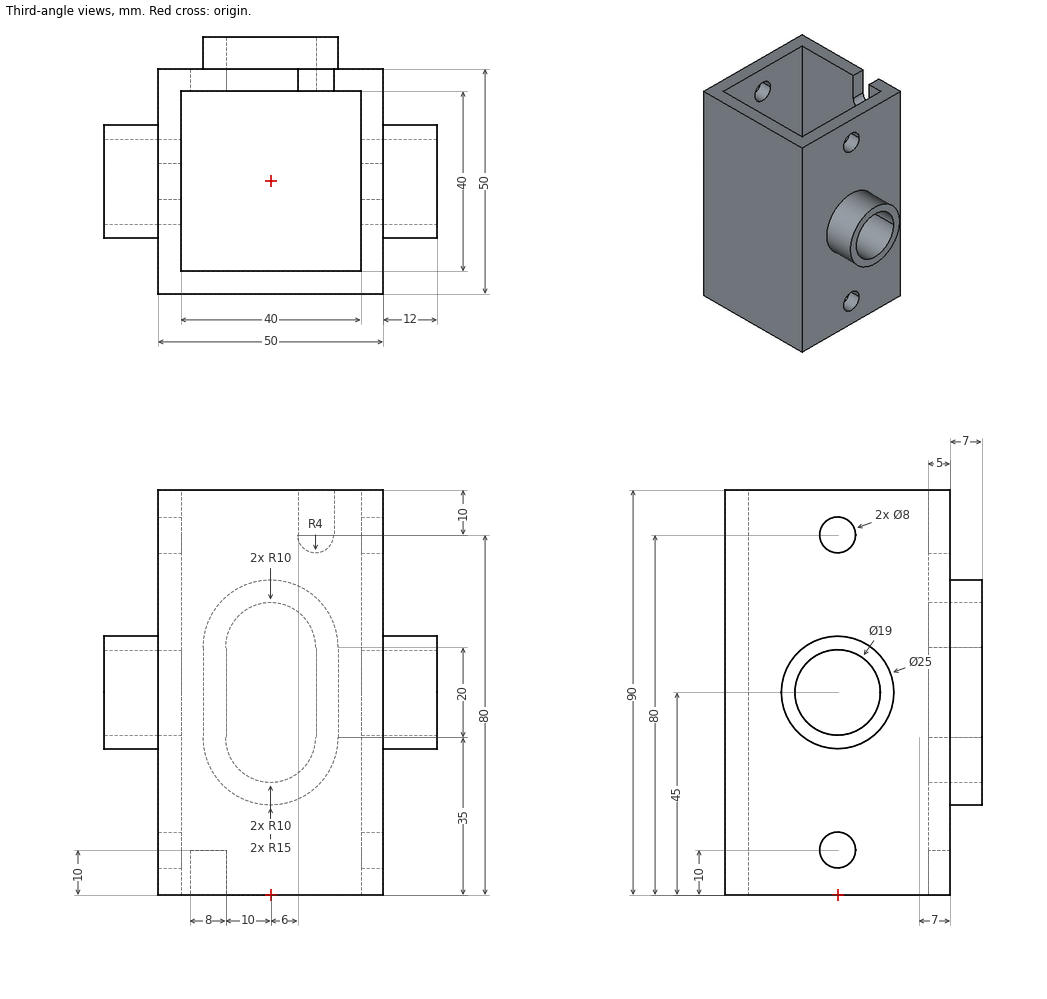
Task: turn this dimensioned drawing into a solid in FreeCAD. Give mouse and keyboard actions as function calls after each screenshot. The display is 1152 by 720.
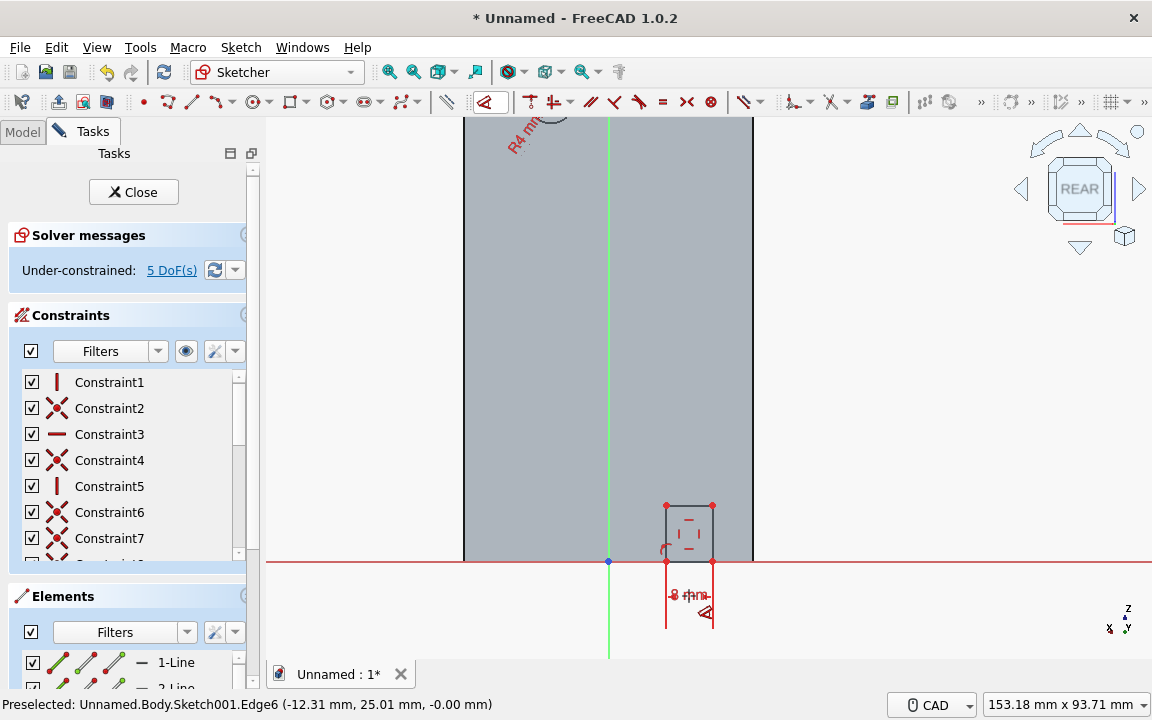
scroll(681, 564, down, 2)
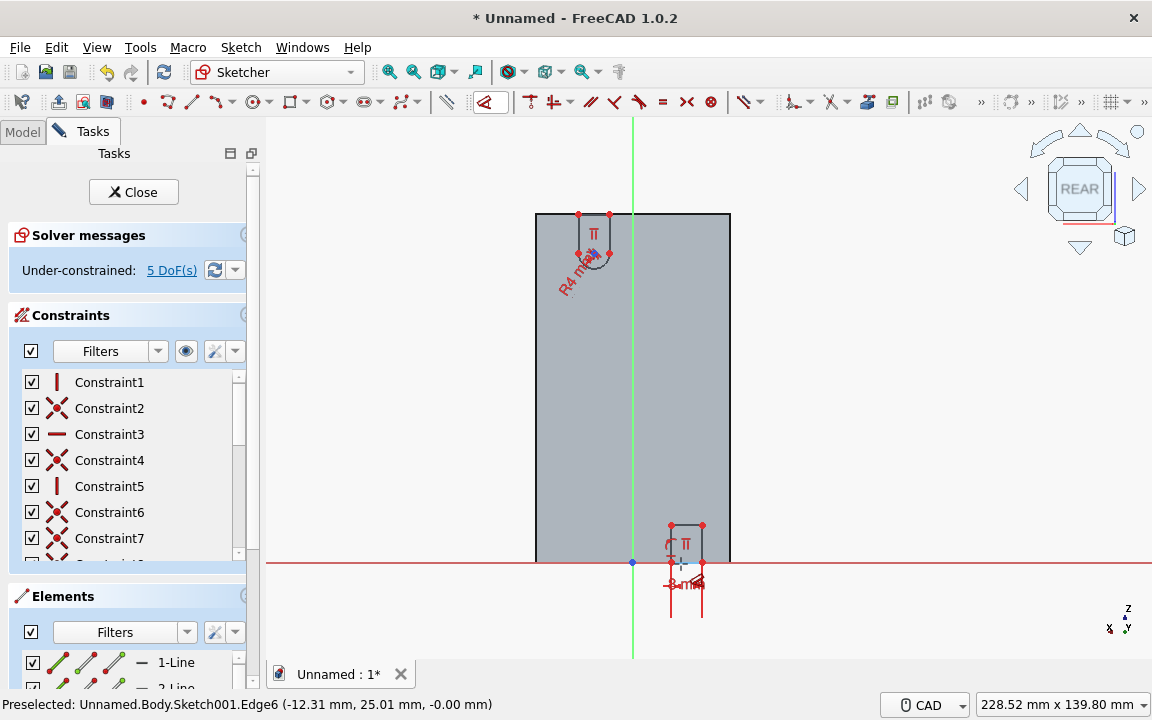
click(610, 242)
click(552, 234)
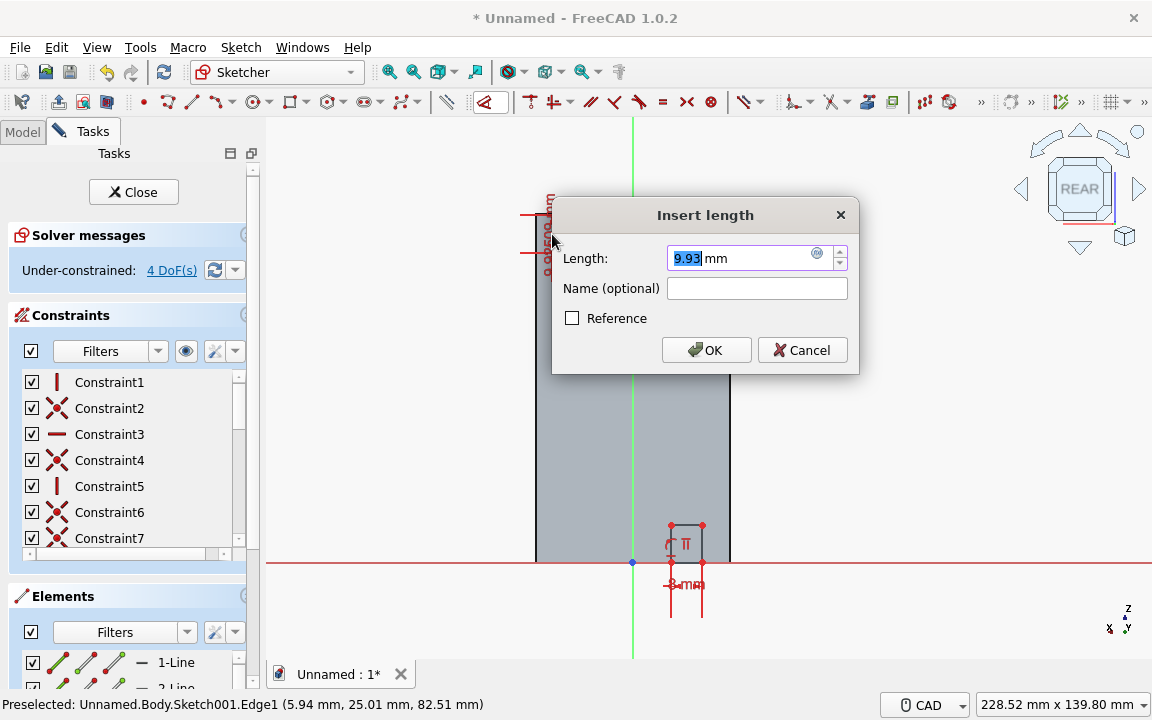
text(10)
key(Return)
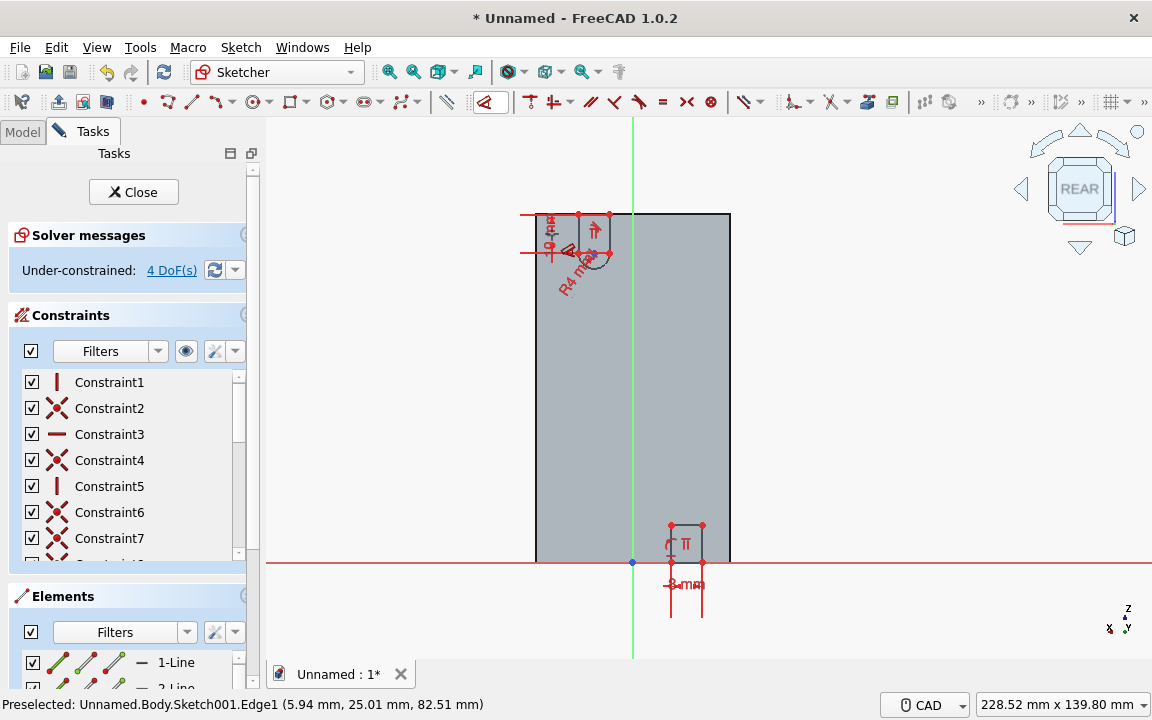
click(671, 536)
click(729, 544)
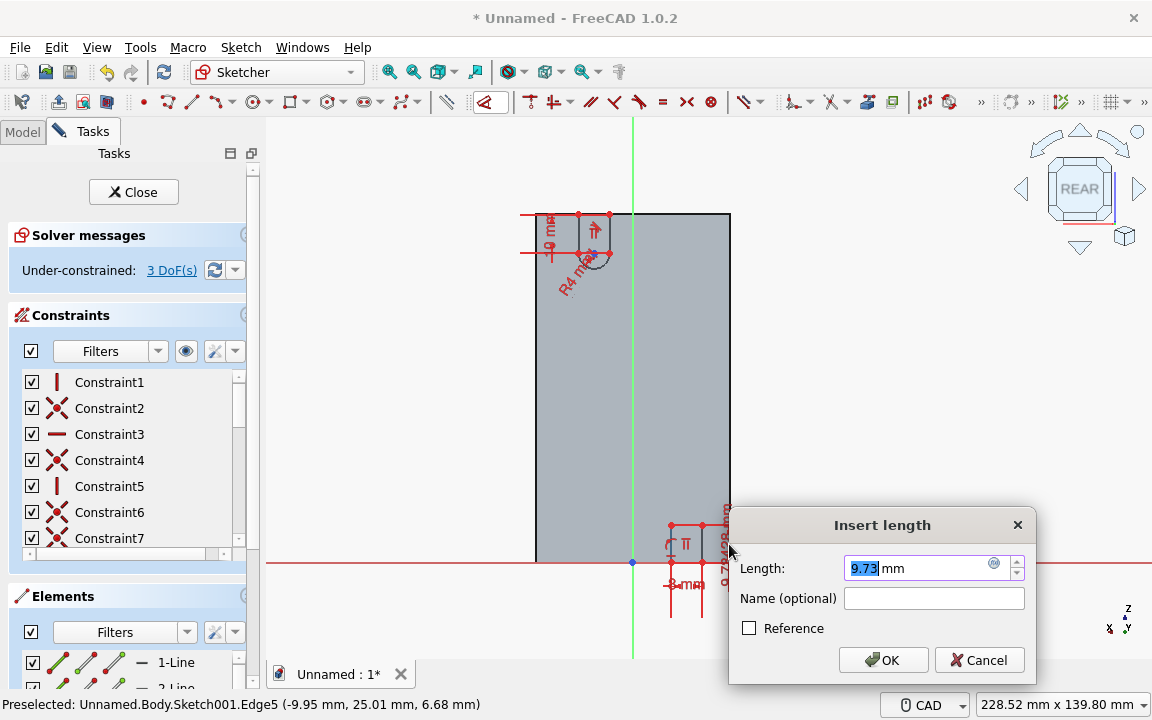
text(10)
key(Return)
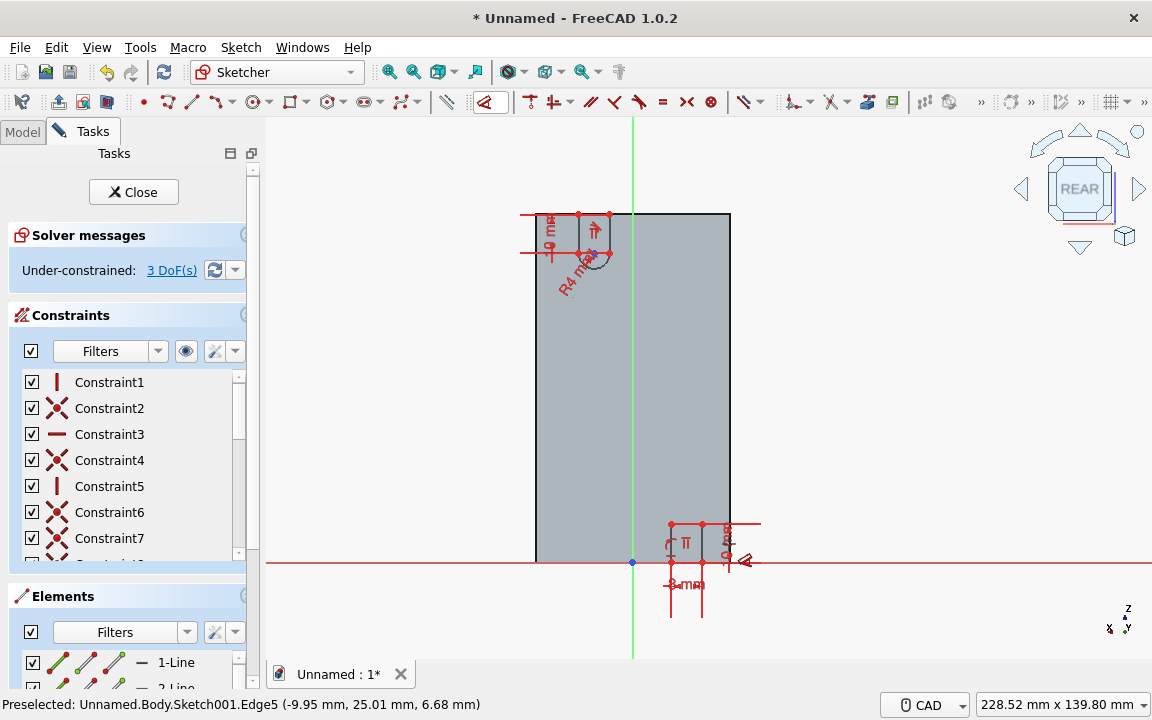
scroll(610, 253, up, 3)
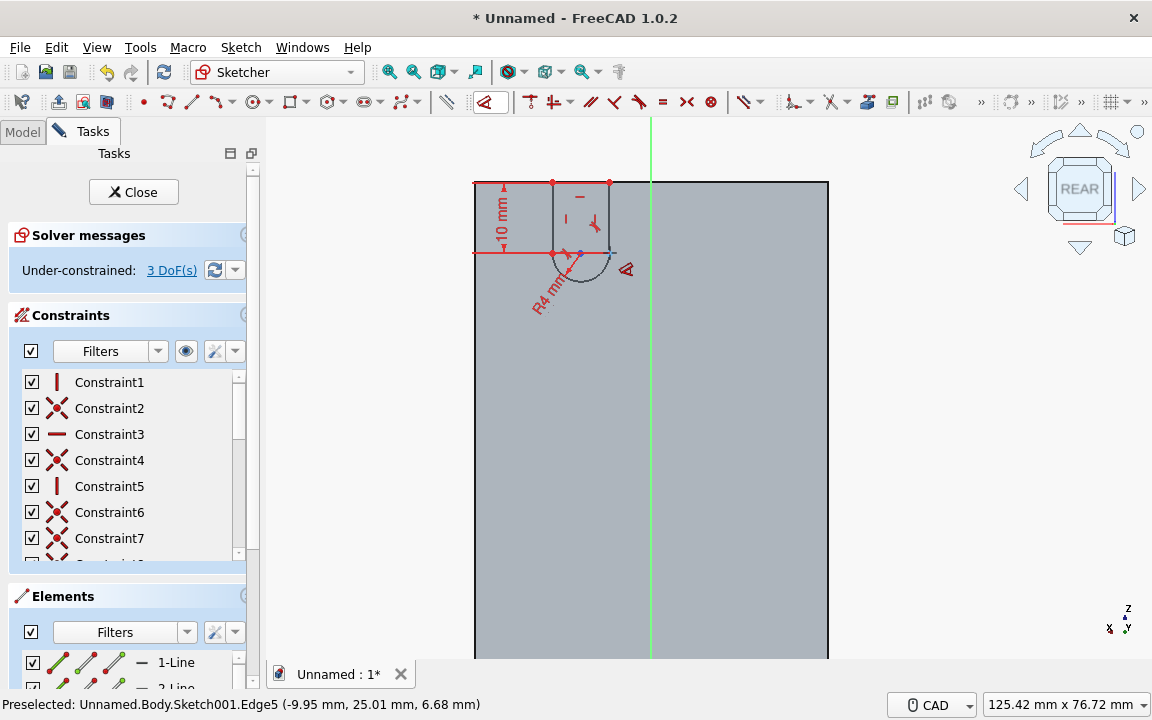
click(609, 253)
click(630, 219)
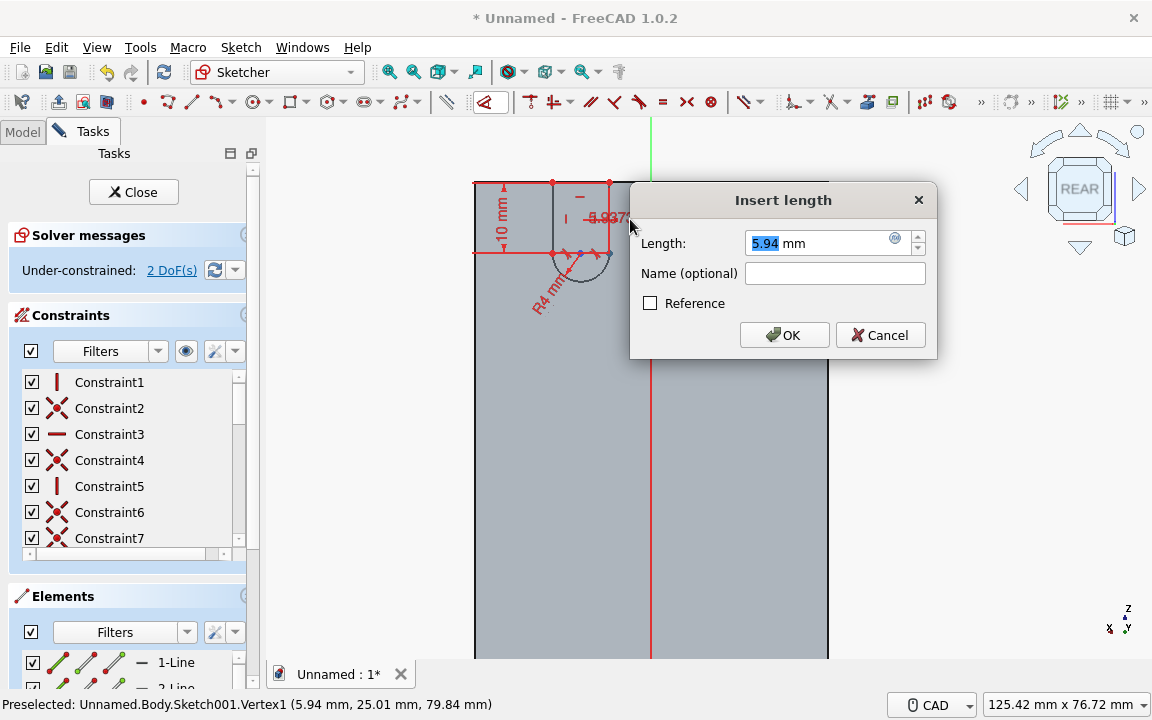
text(6)
key(Return)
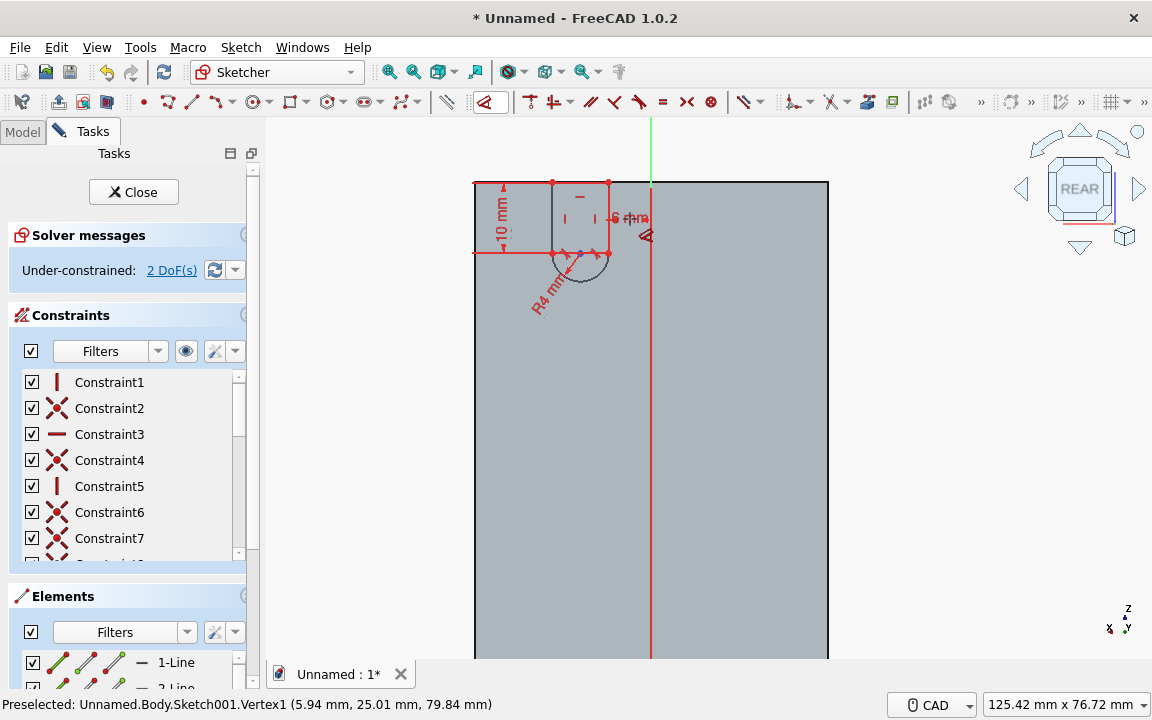
click(609, 253)
click(575, 442)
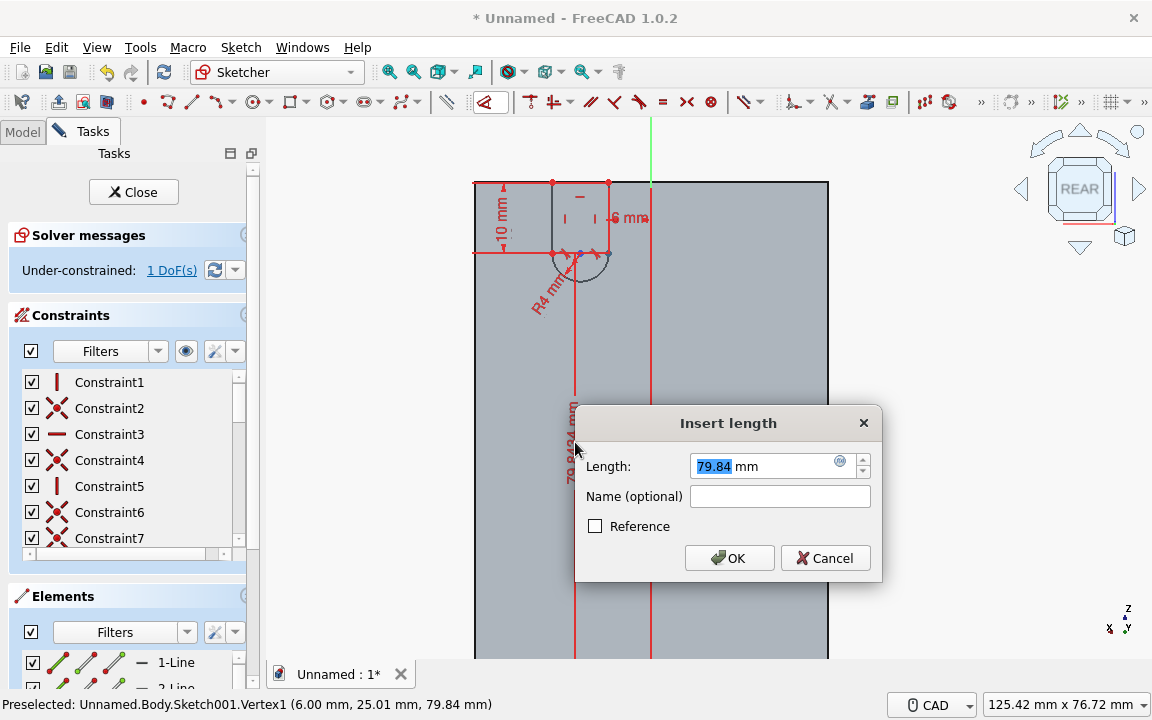
text(80)
key(Return)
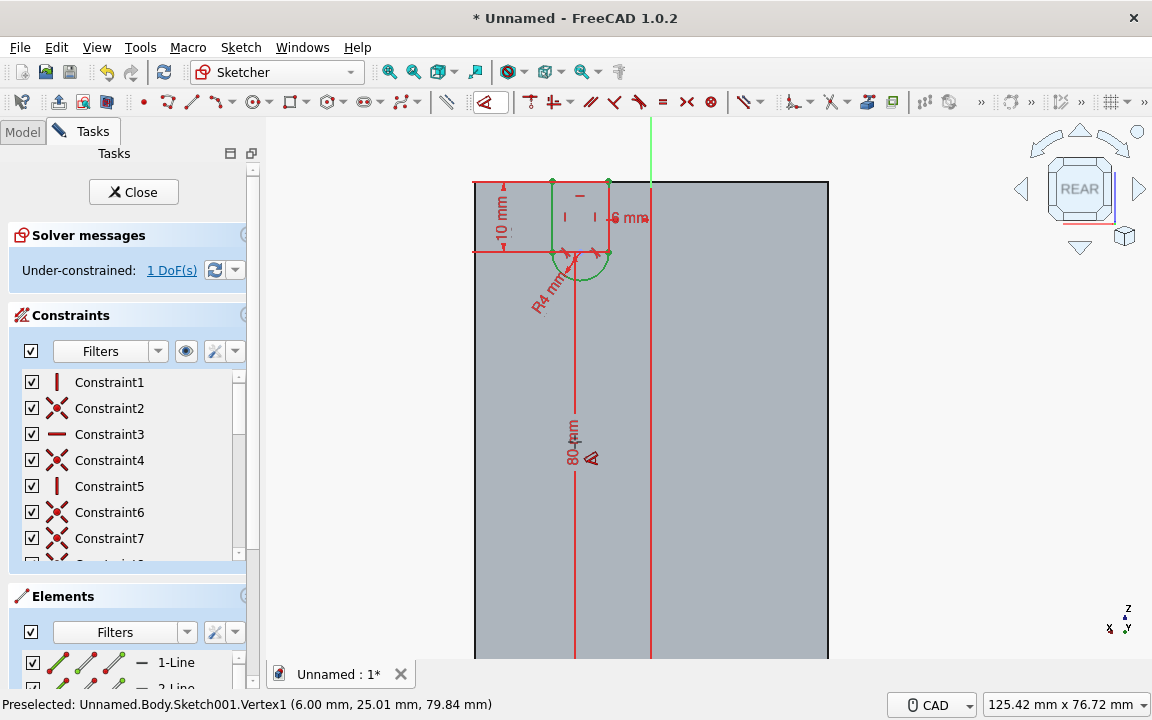
scroll(610, 252, down, 3)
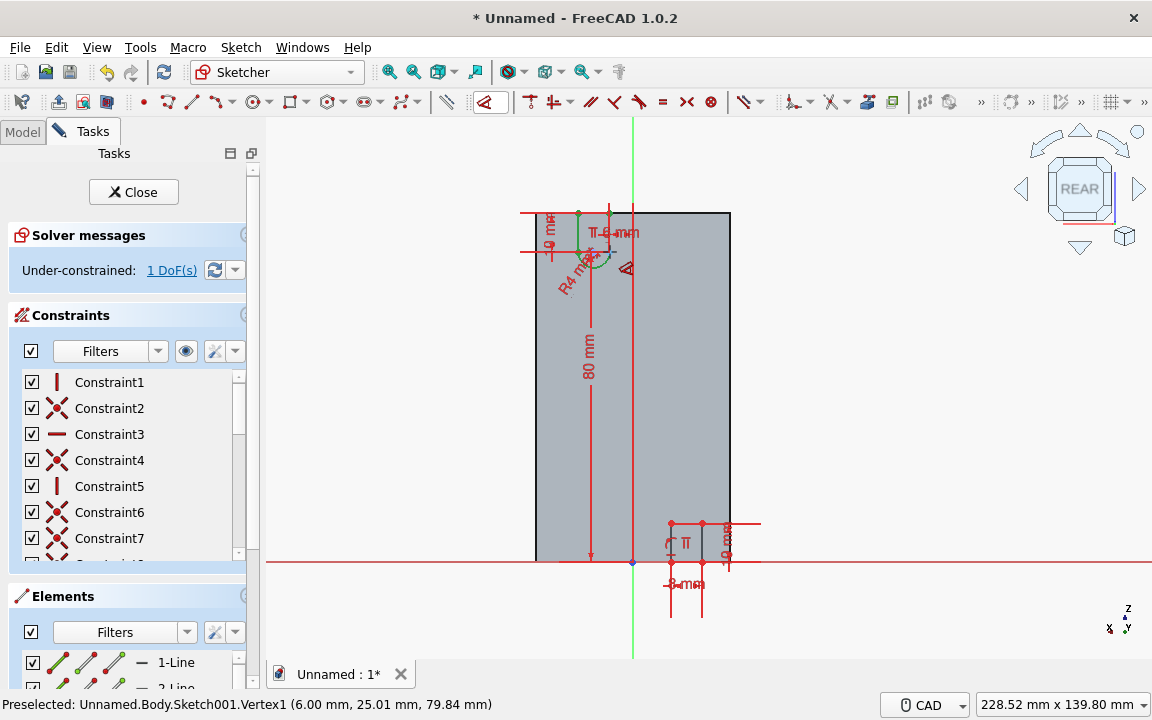
click(671, 524)
click(652, 490)